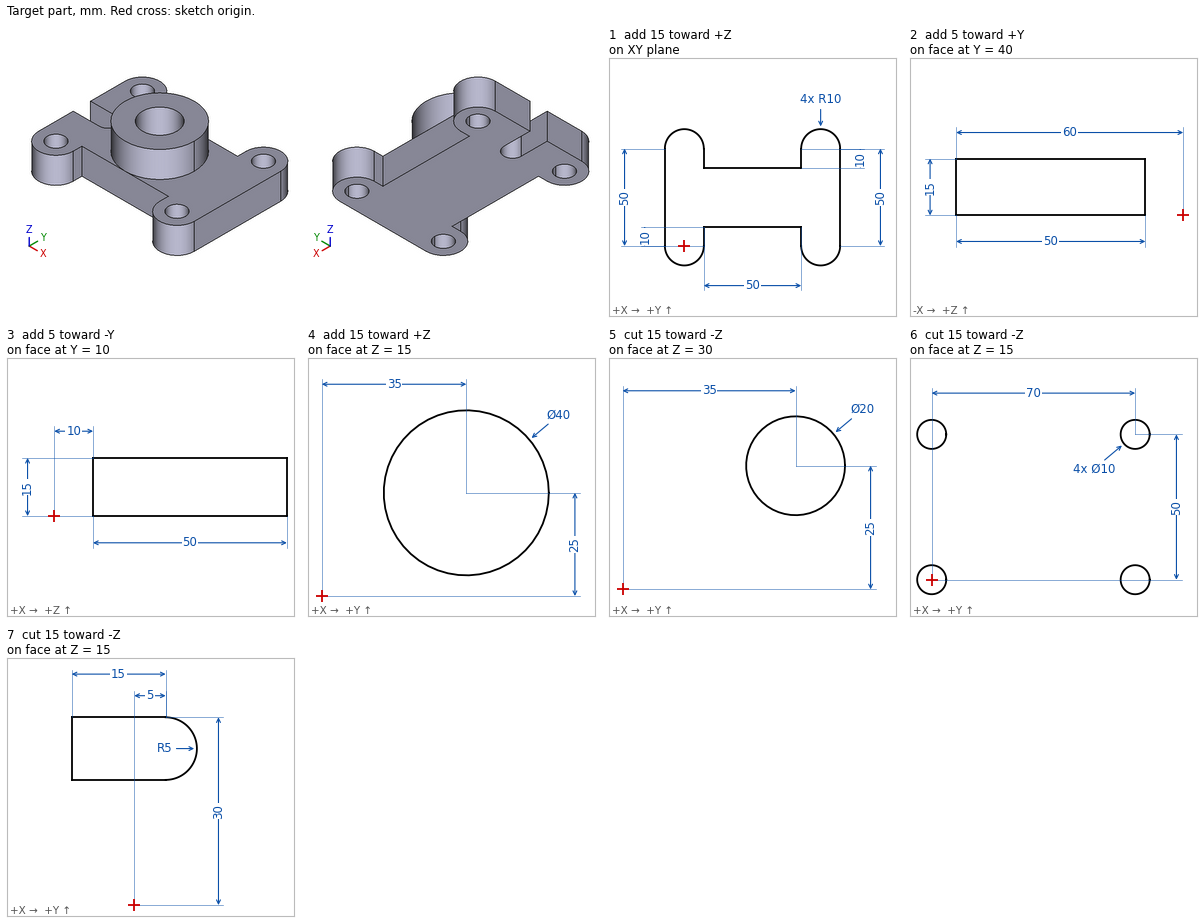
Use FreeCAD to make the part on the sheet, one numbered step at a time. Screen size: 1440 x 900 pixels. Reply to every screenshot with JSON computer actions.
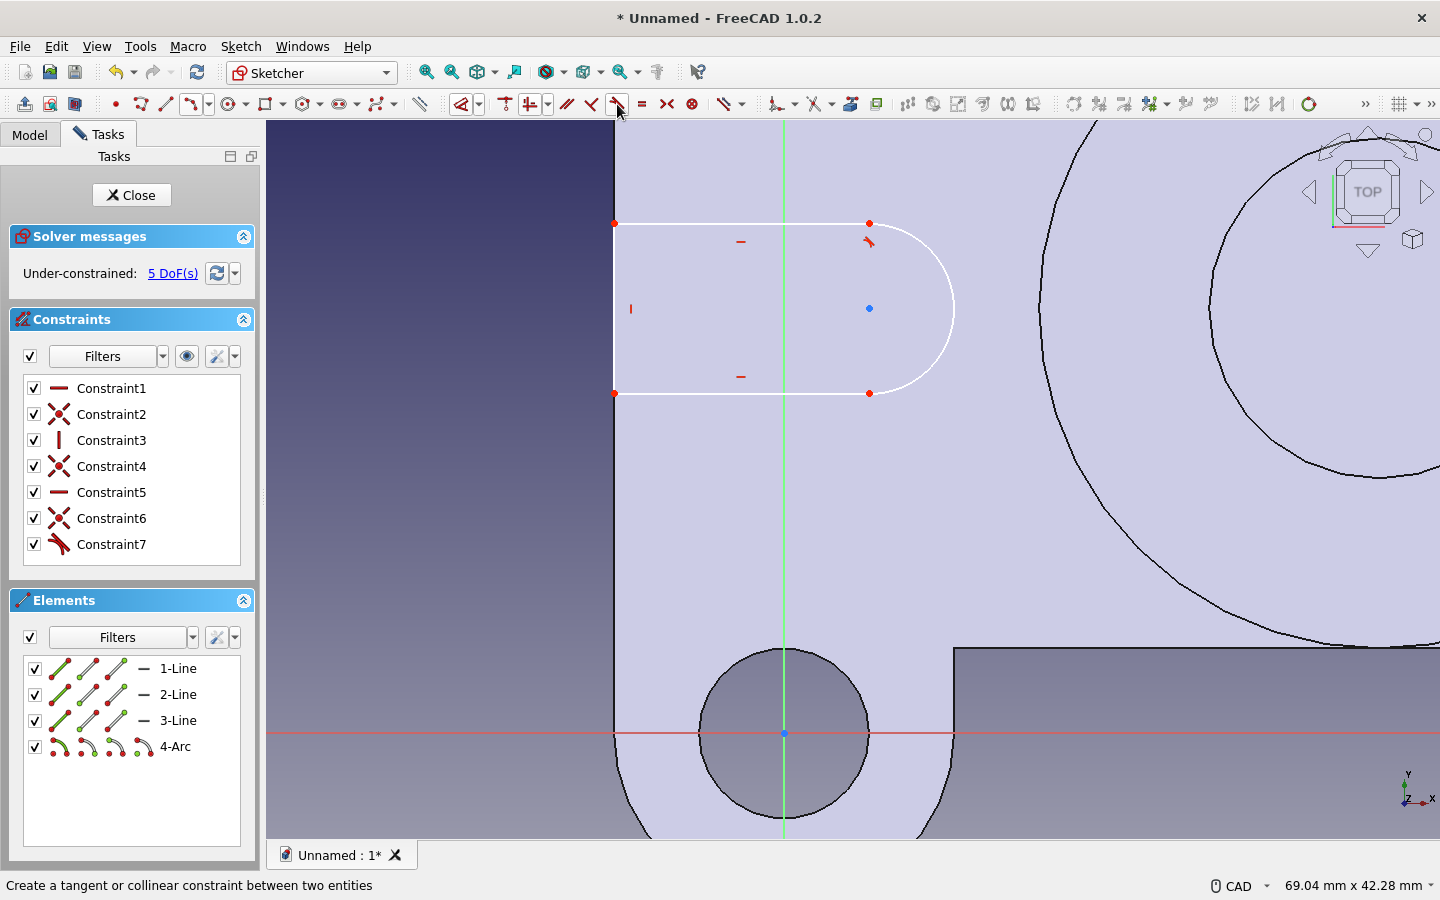
{"action": "left_click", "coordinate": [690, 394]}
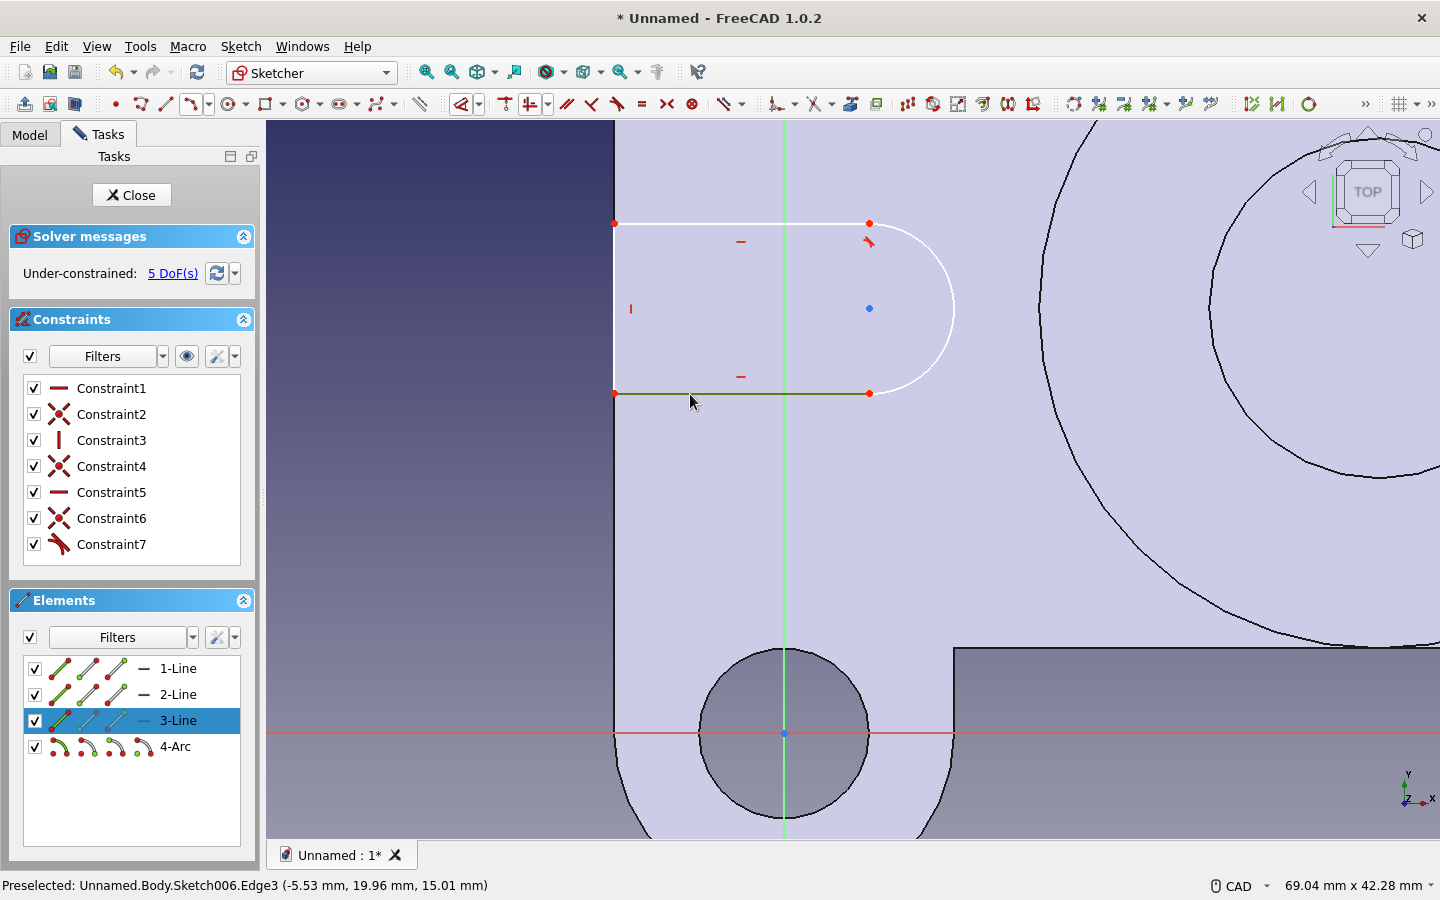
{"action": "left_click", "coordinate": [938, 359]}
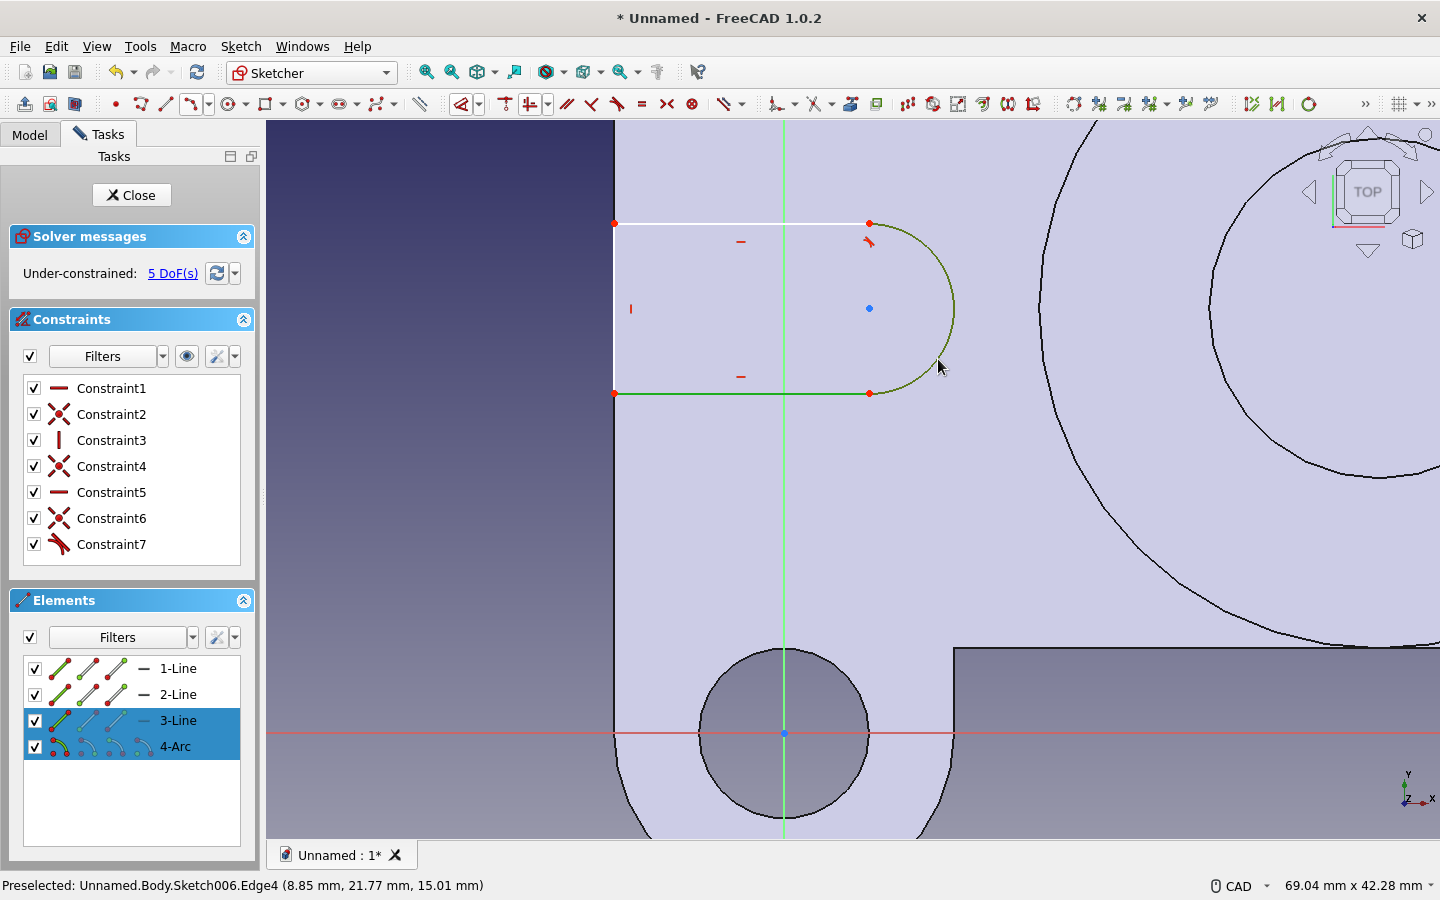
{"action": "left_click", "coordinate": [617, 104]}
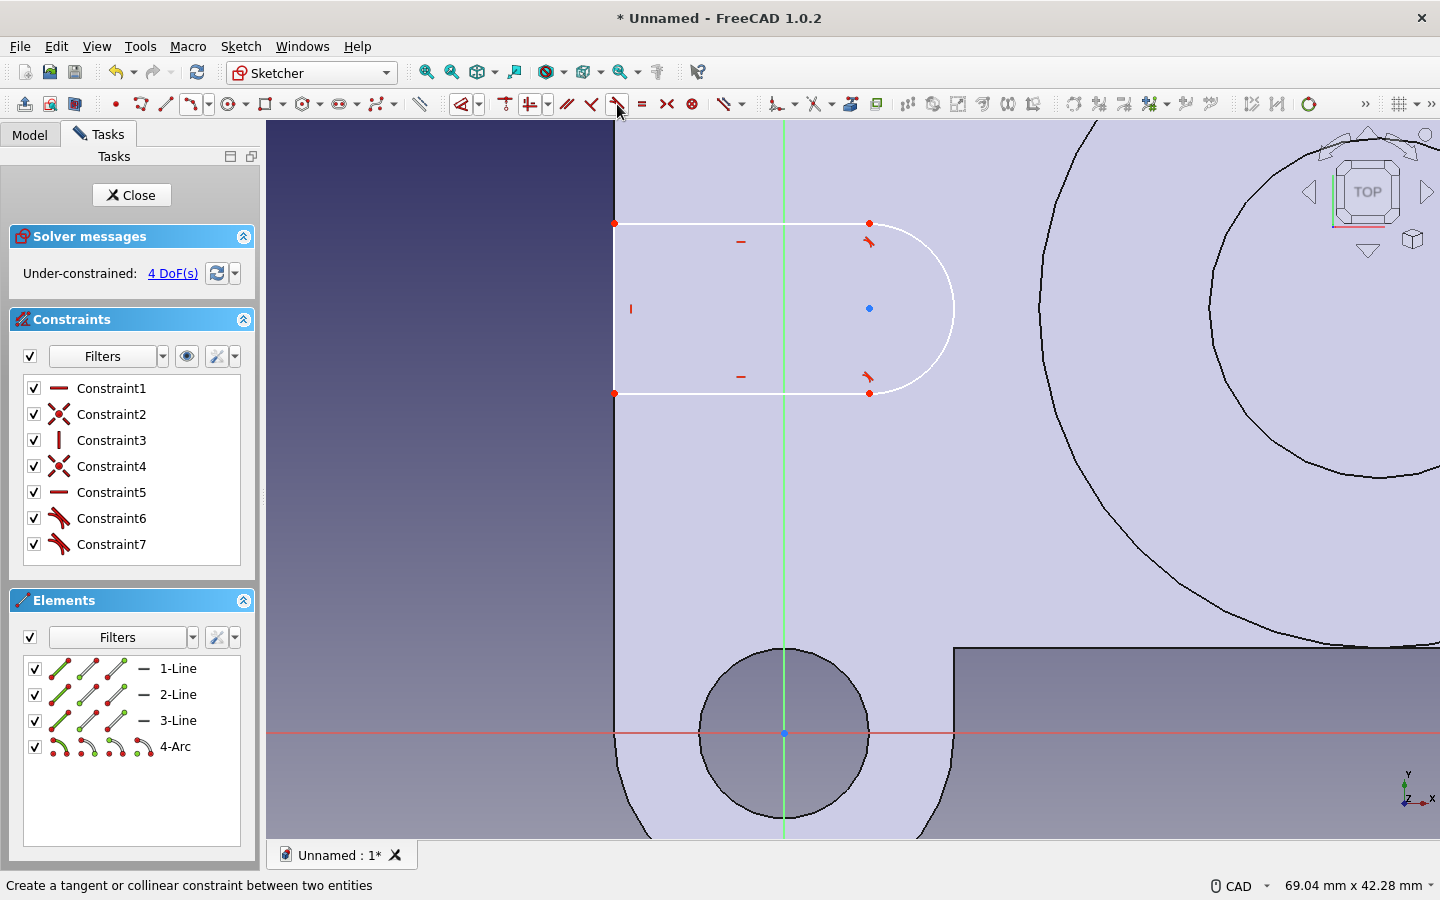
{"action": "left_click", "coordinate": [938, 359]}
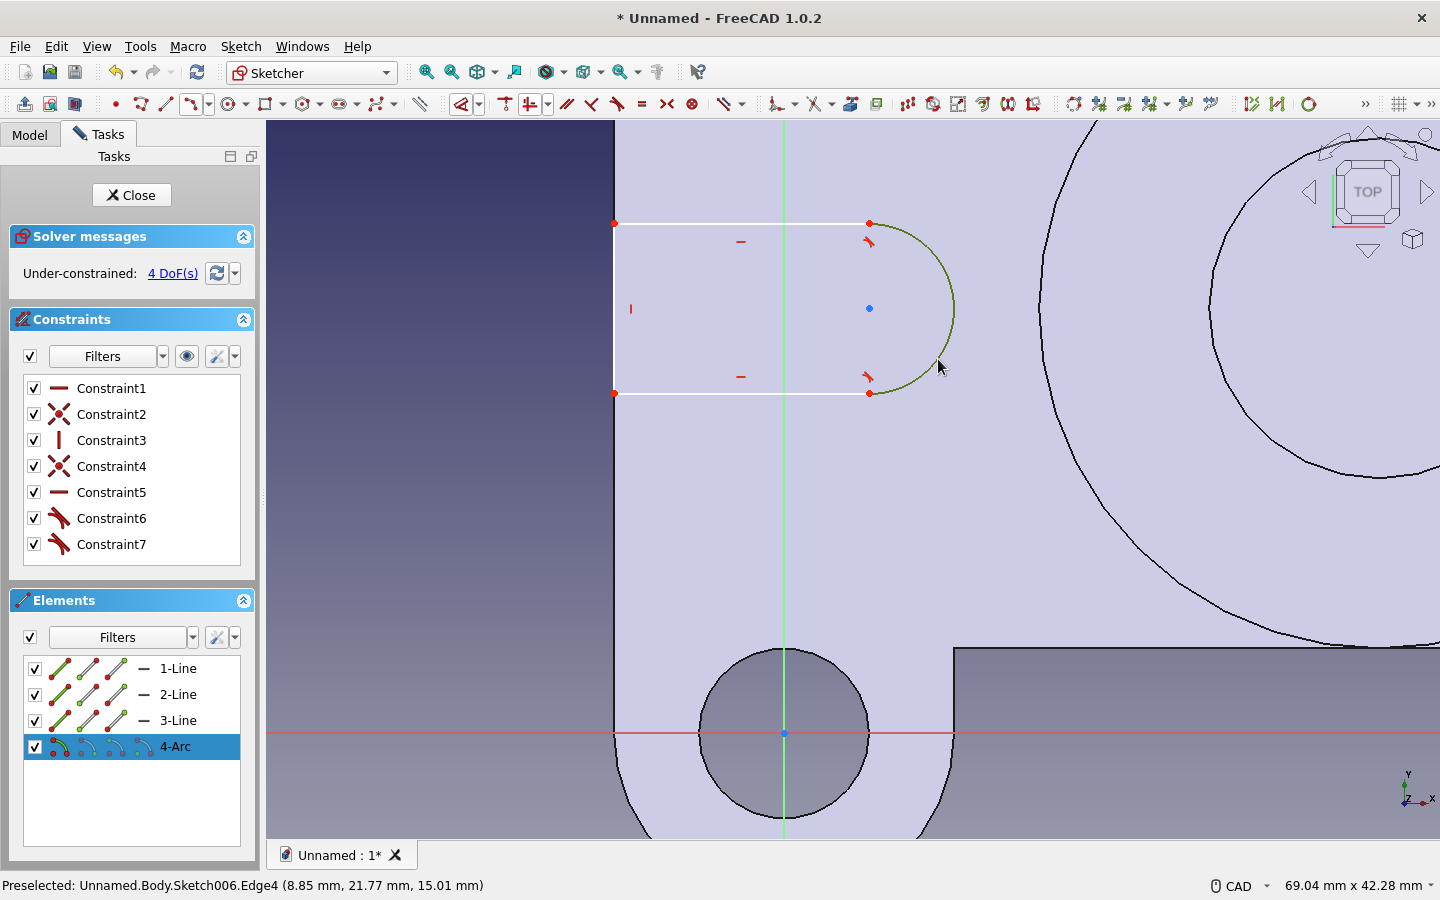
{"action": "left_click", "coordinate": [478, 104]}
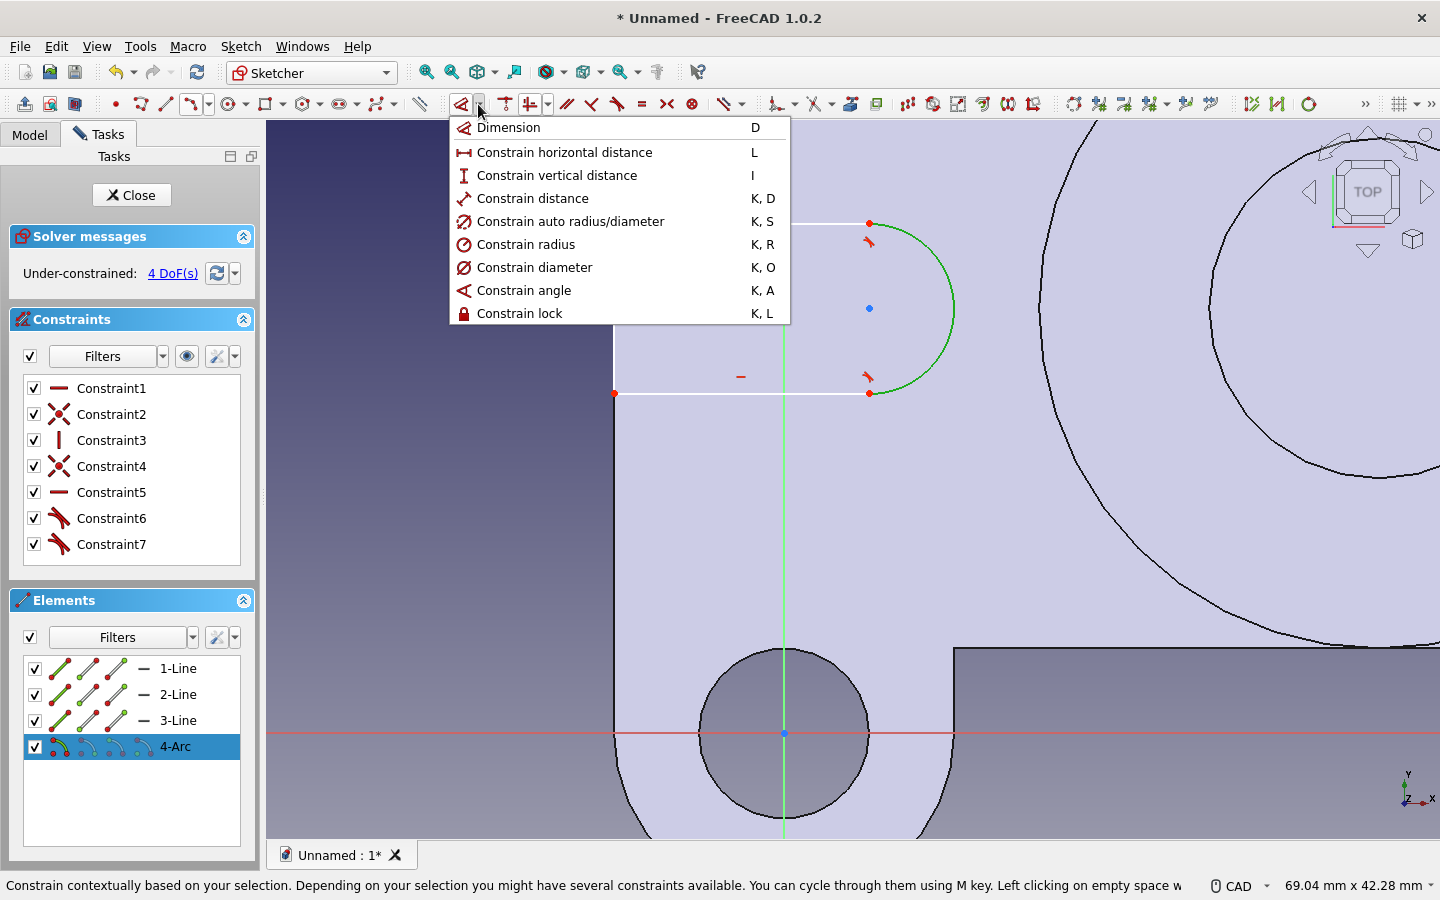
{"action": "left_click", "coordinate": [620, 244]}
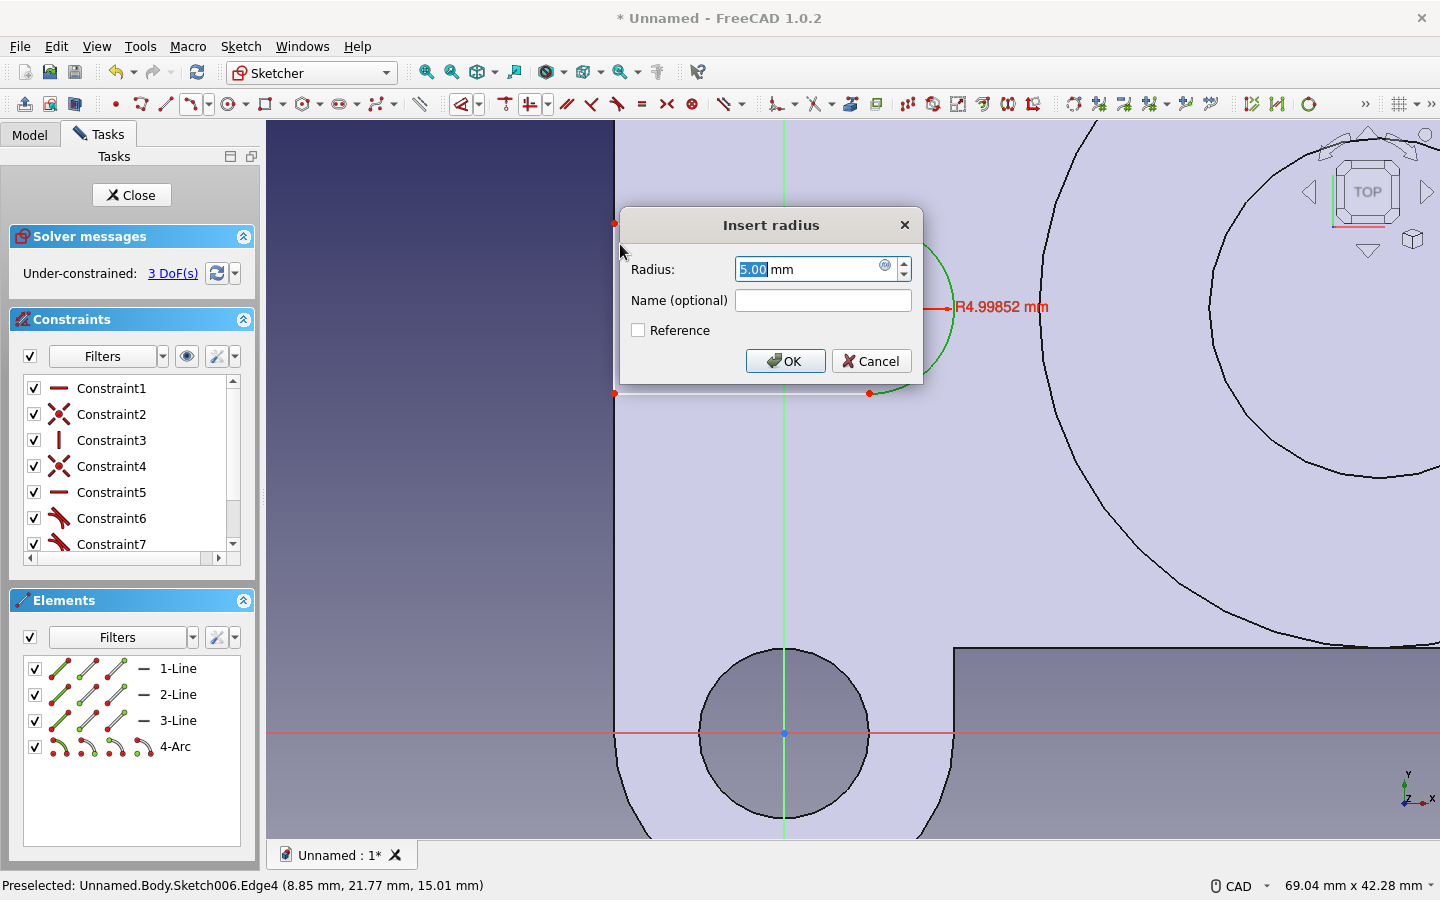
{"action": "type", "text": "5"}
{"action": "key", "text": "Return"}